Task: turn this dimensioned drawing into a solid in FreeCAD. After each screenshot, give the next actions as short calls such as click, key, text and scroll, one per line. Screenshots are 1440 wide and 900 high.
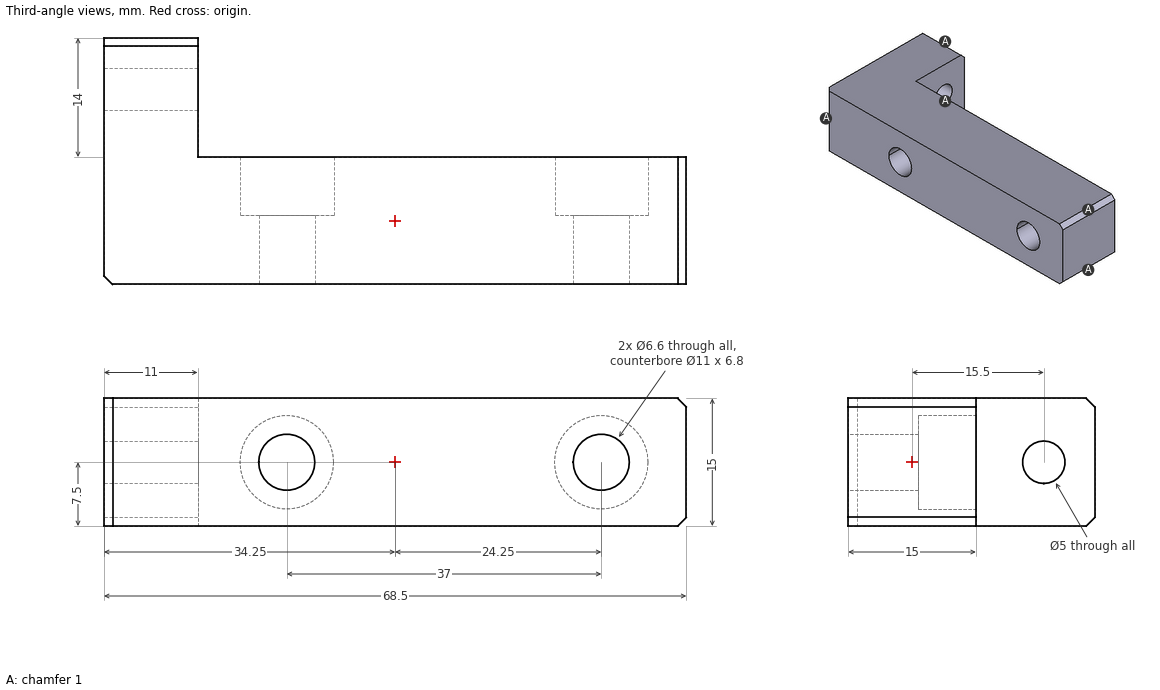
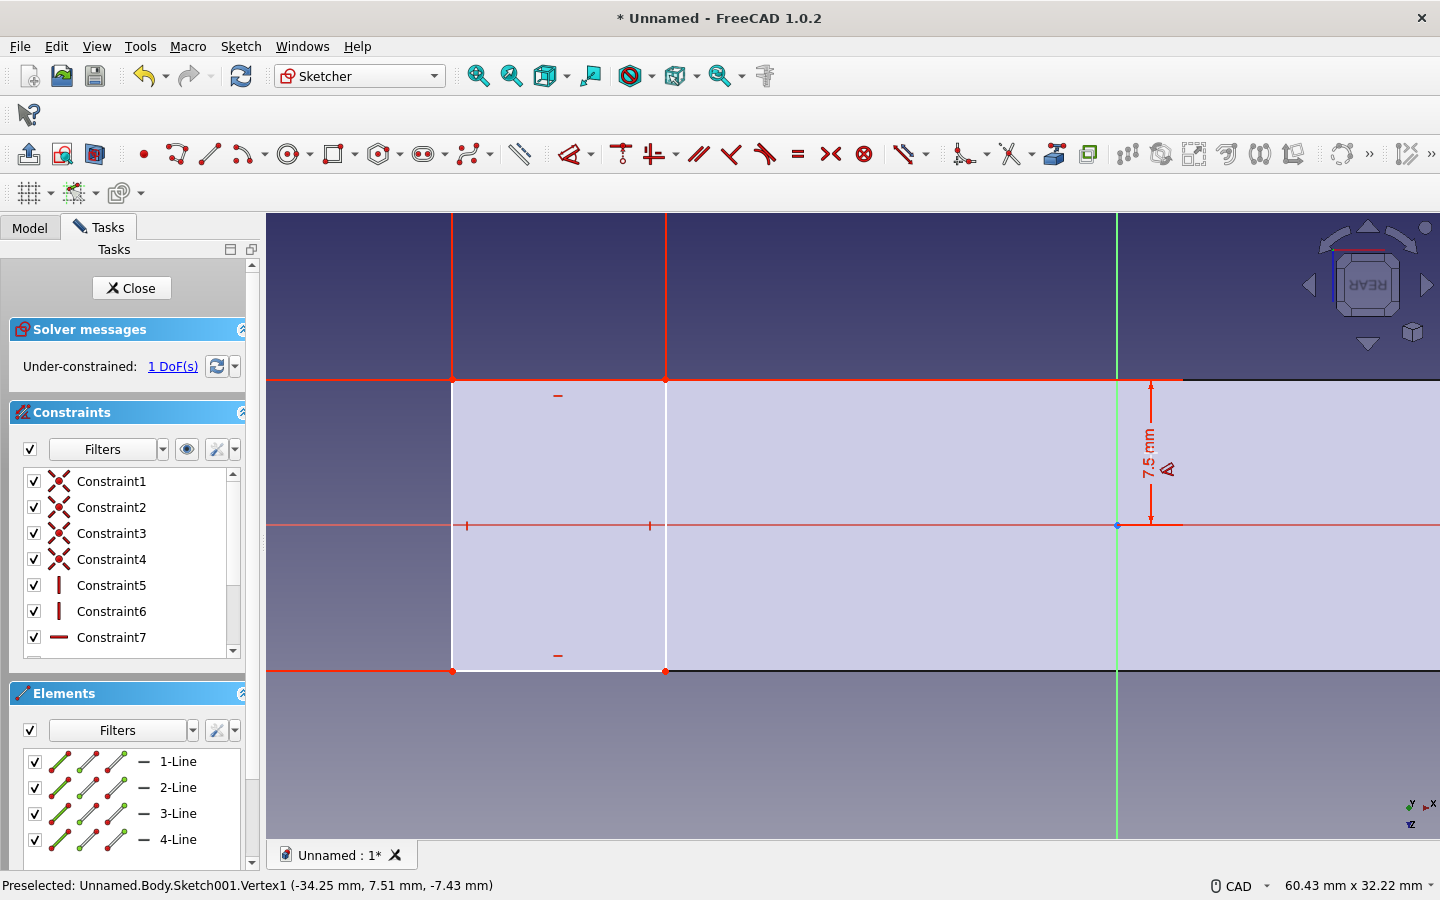
click(452, 380)
click(785, 346)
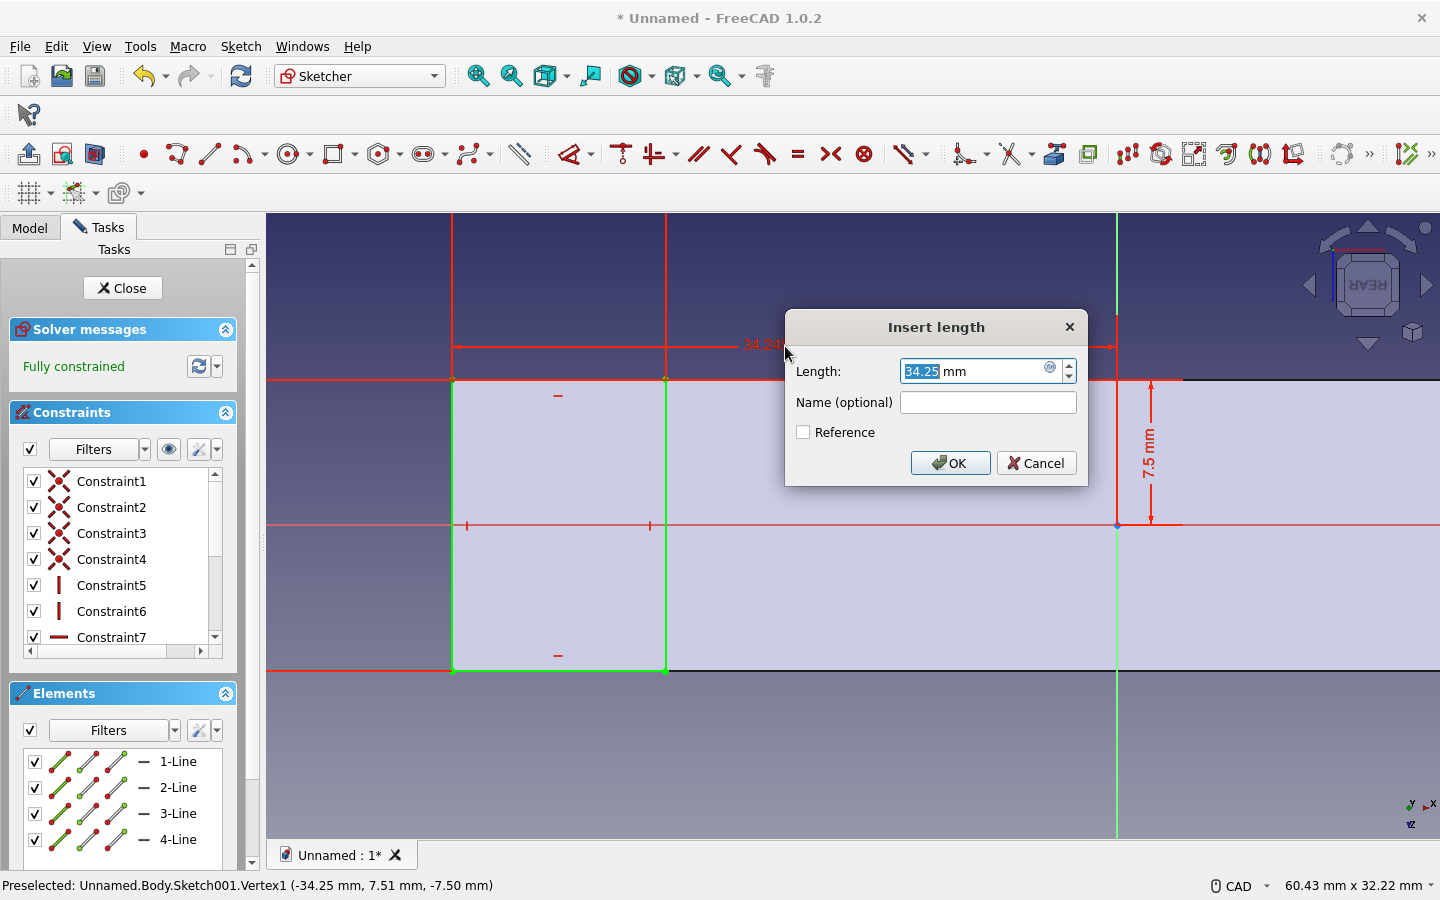
text(34.25)
key(Return)
key(Escape)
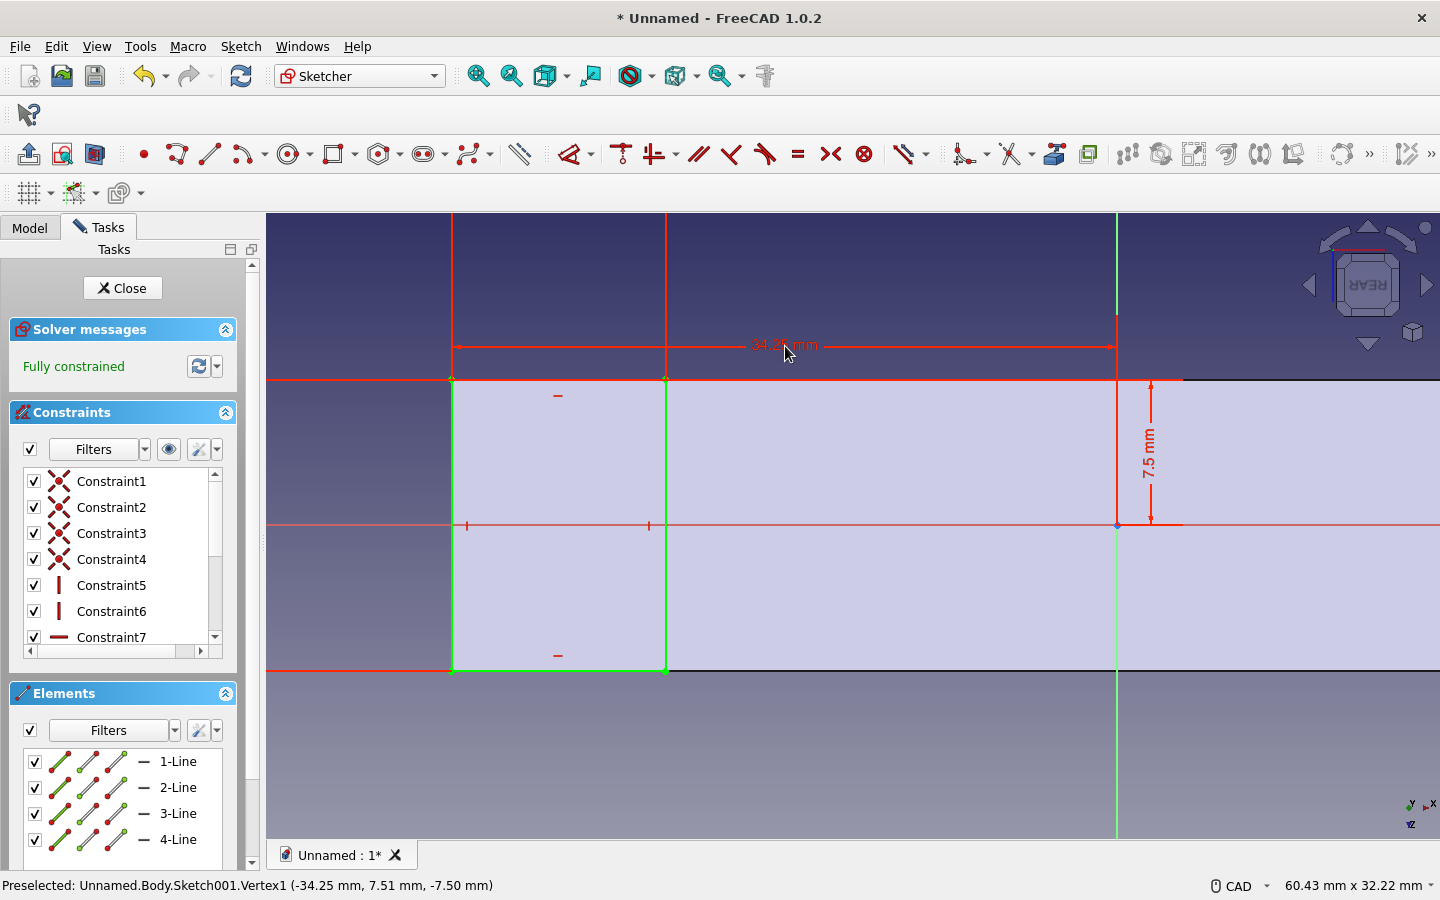
click(123, 288)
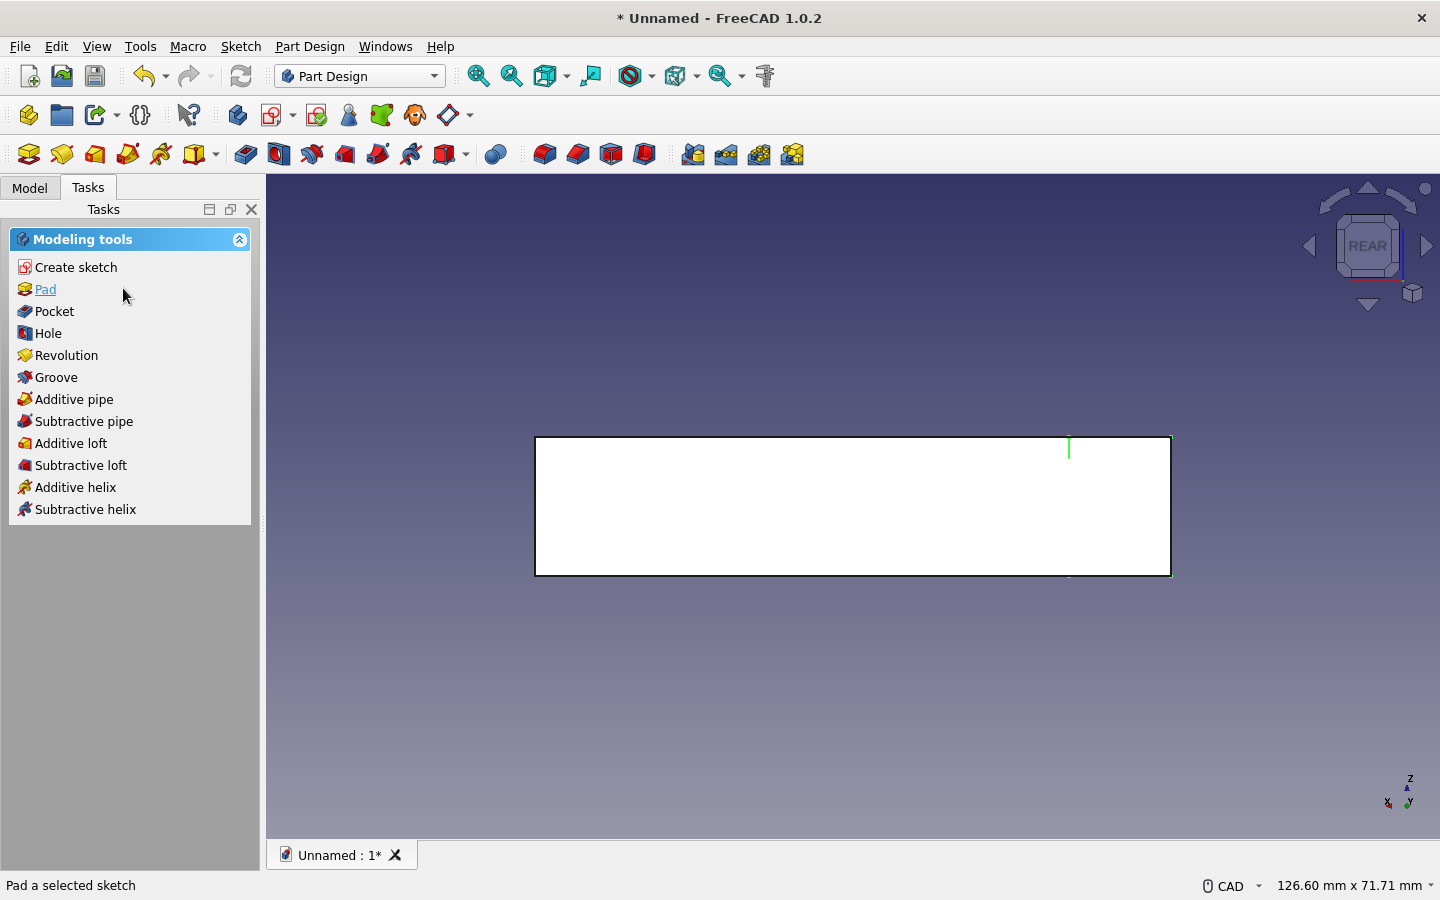
click(29, 154)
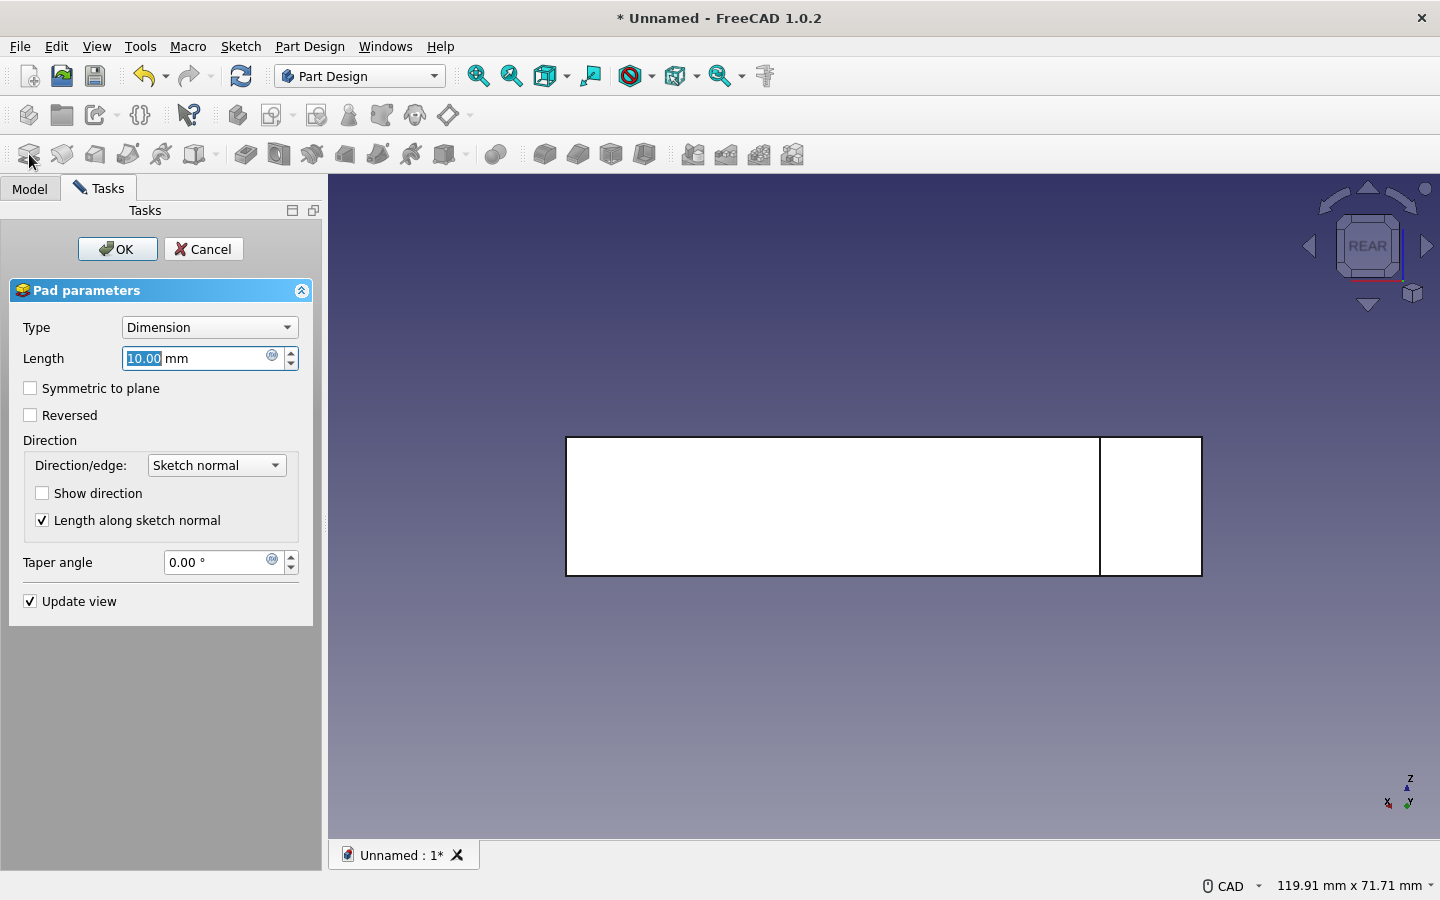
text(14)
key(Tab)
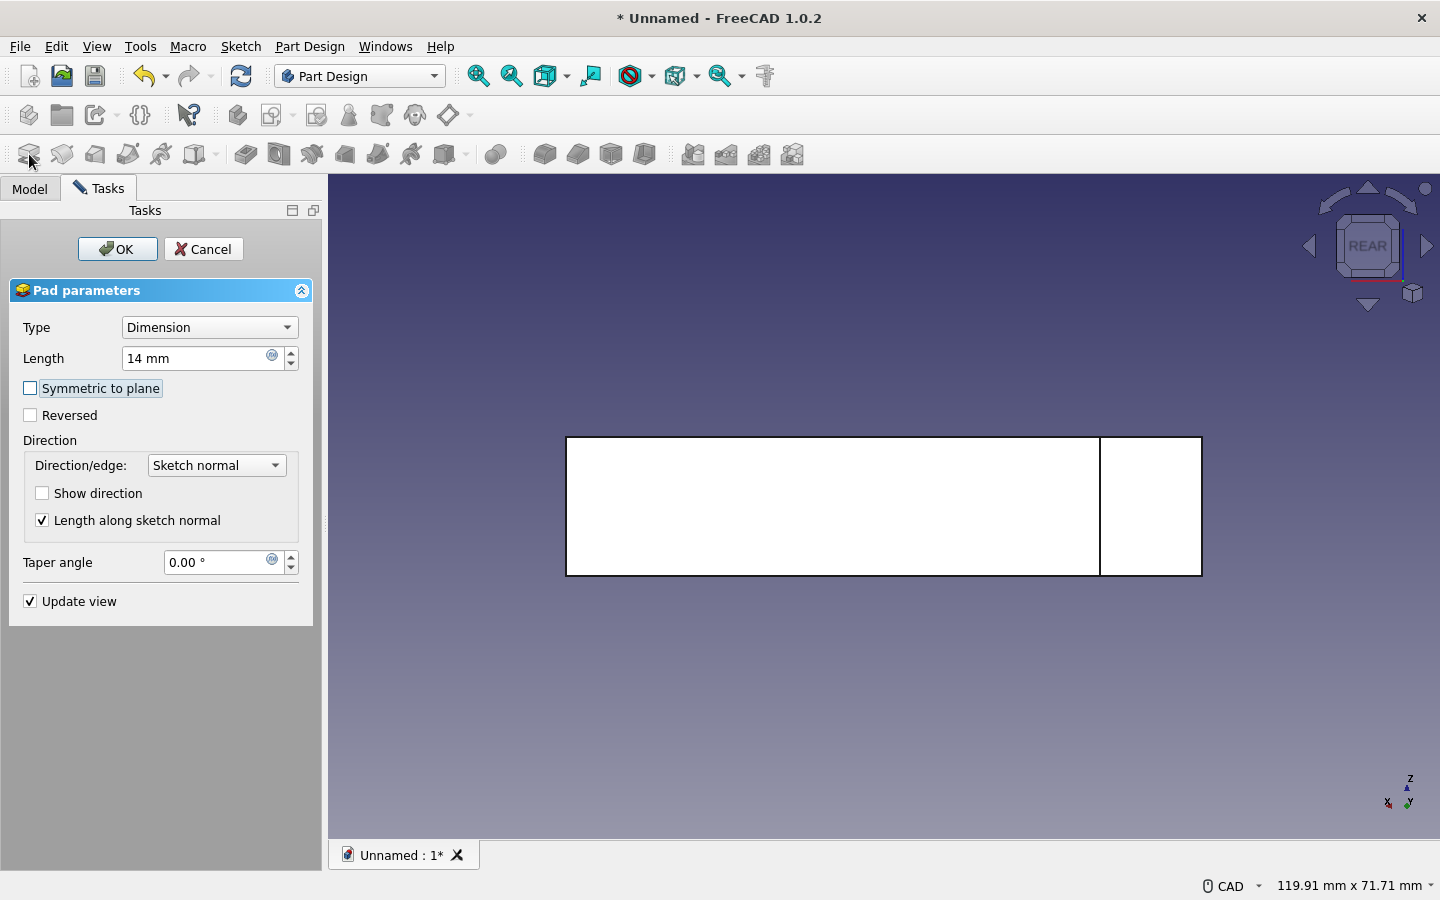
click(118, 249)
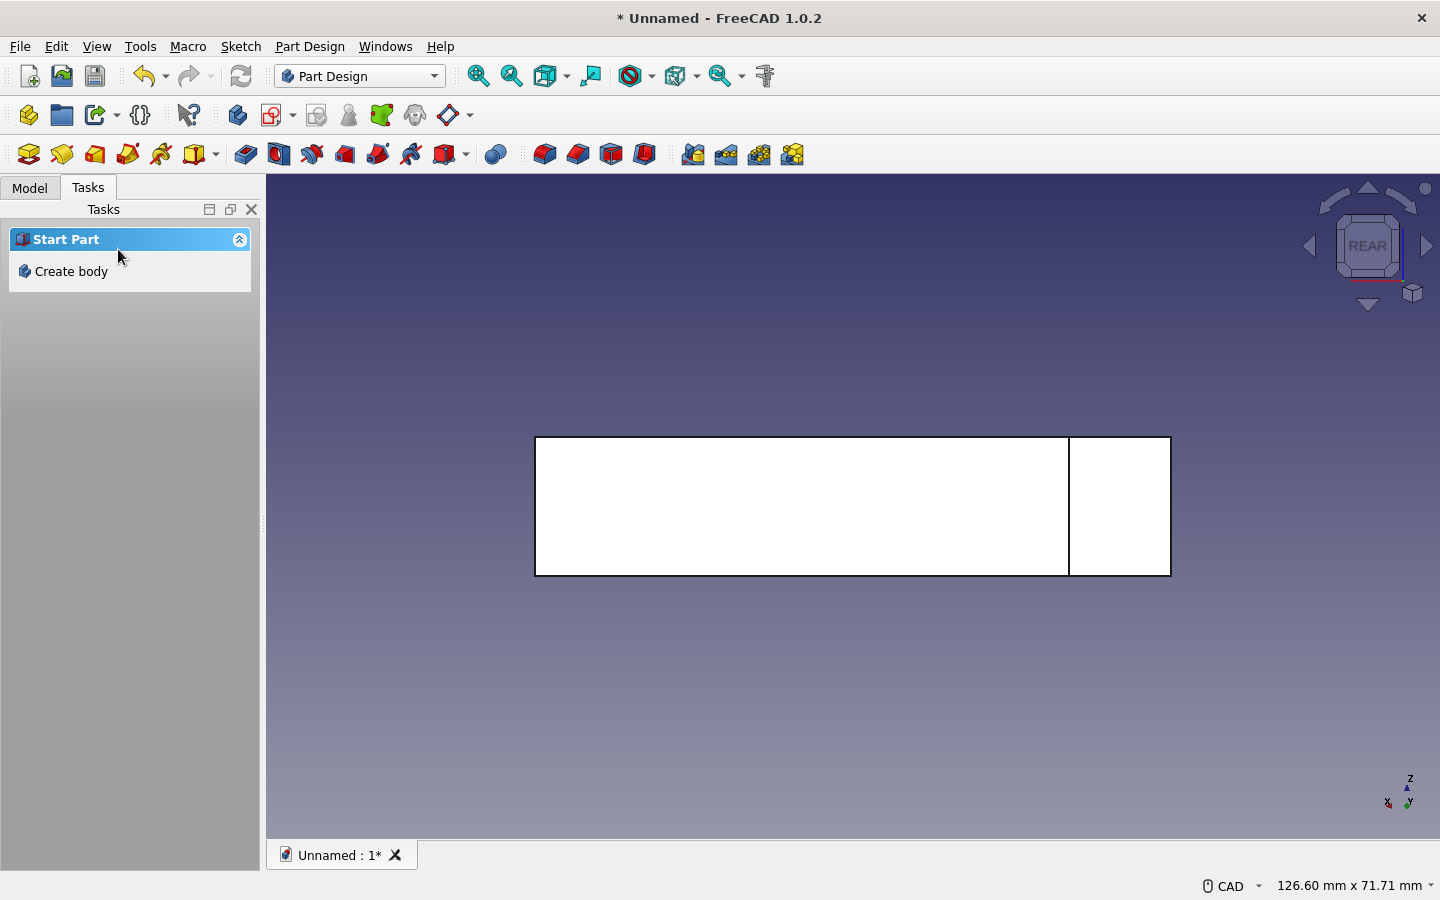
click(1120, 575)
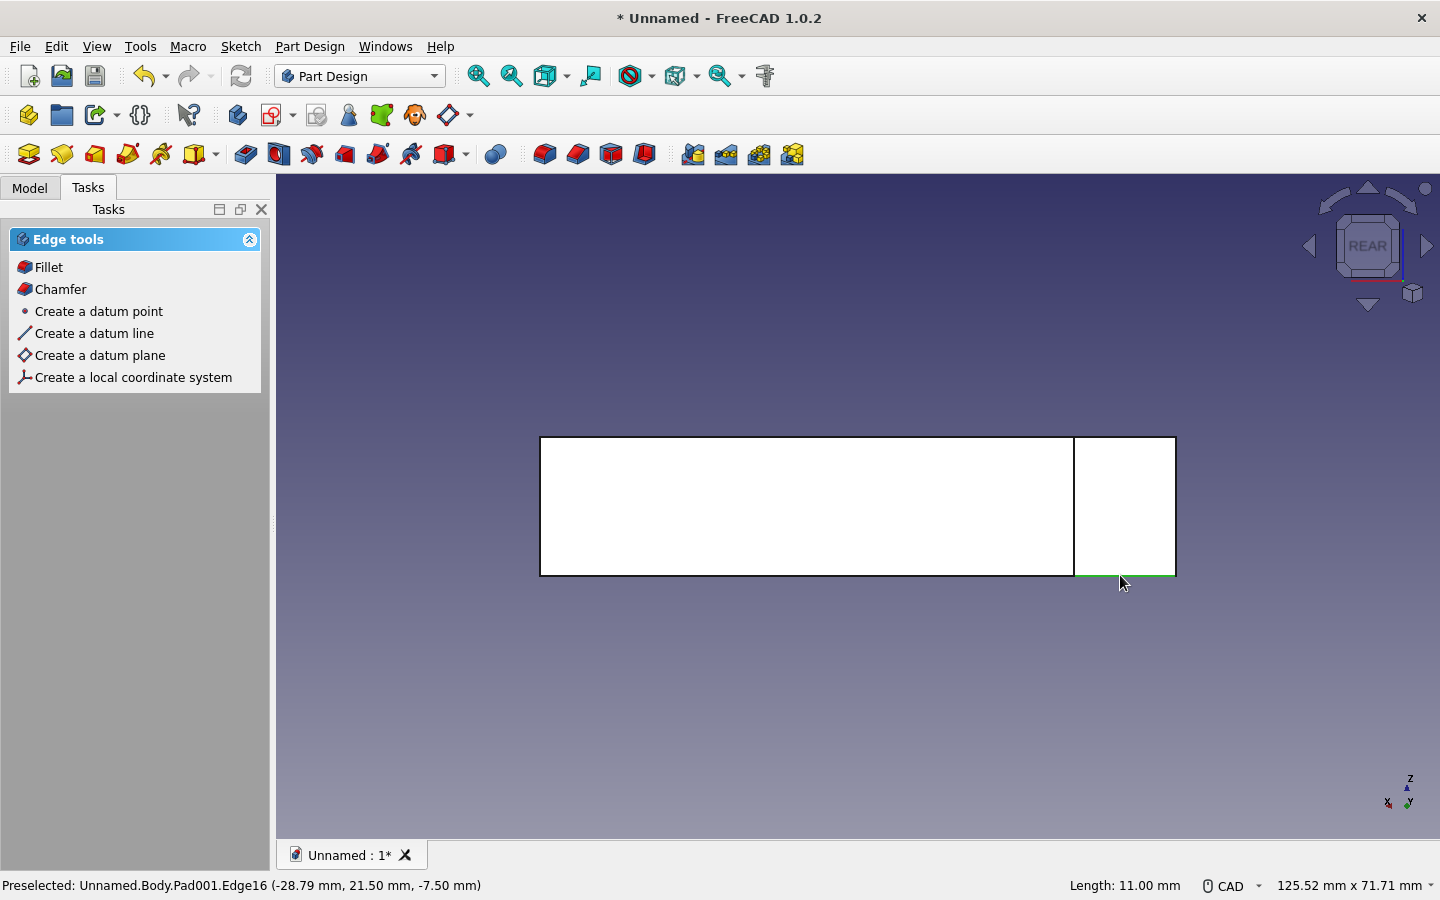
key(0)